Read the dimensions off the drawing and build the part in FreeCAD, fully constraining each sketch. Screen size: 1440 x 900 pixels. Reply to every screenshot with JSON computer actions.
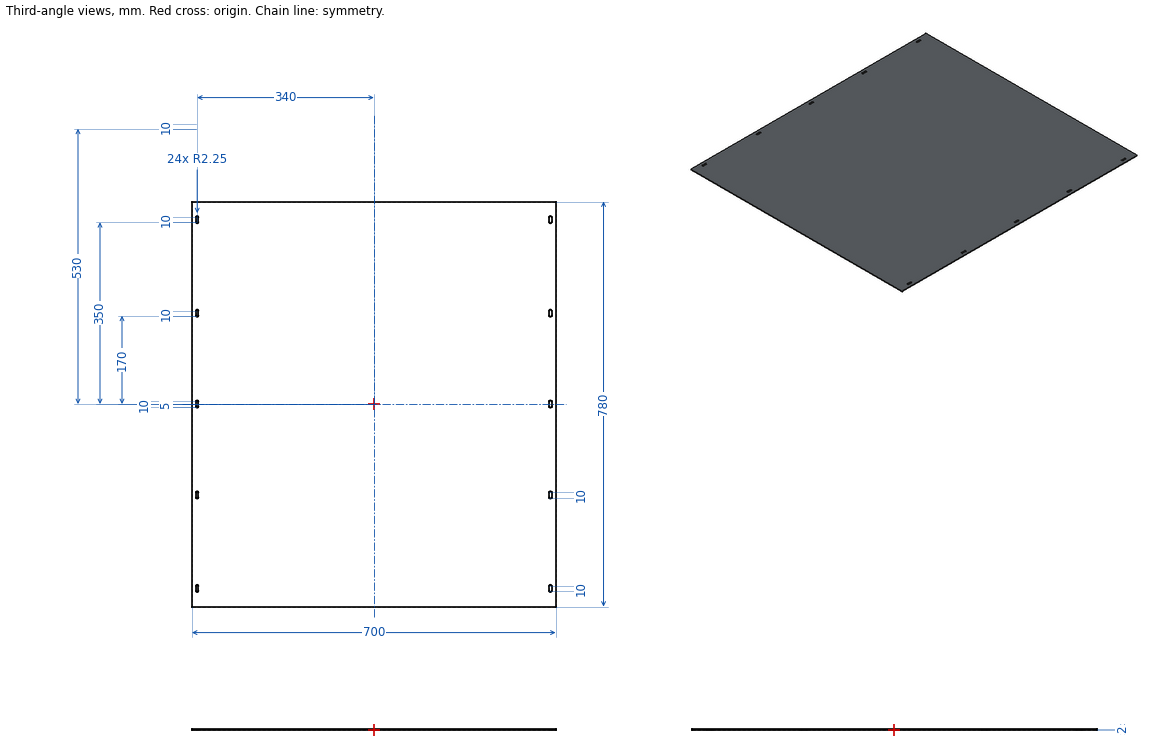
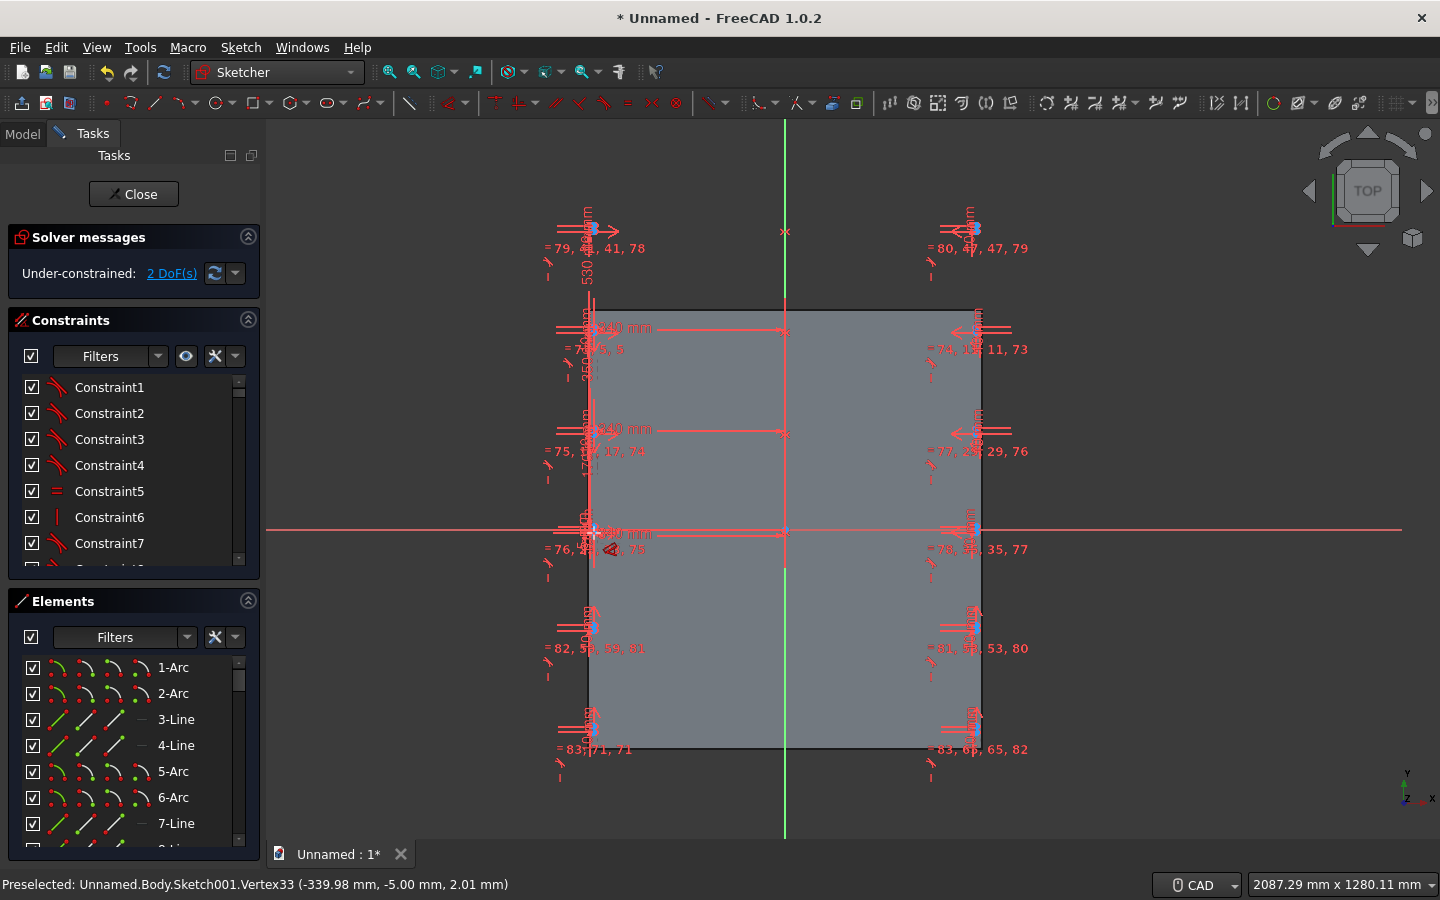
{"action": "scroll", "coordinate": [594, 232], "scroll_direction": "up", "scroll_amount": 12}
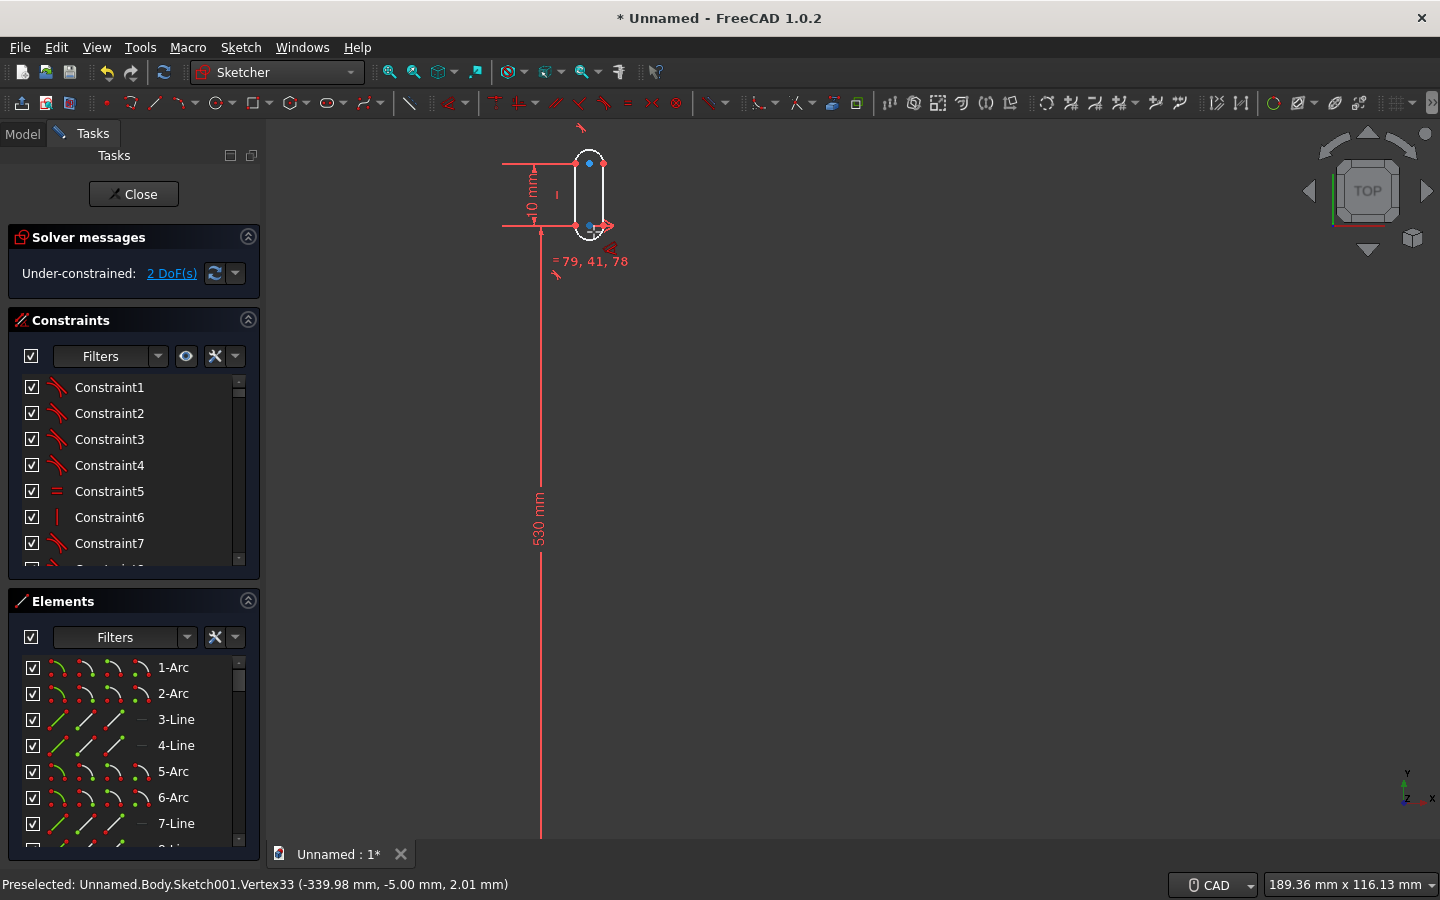
{"action": "left_click", "coordinate": [589, 226]}
{"action": "left_click", "coordinate": [932, 192]}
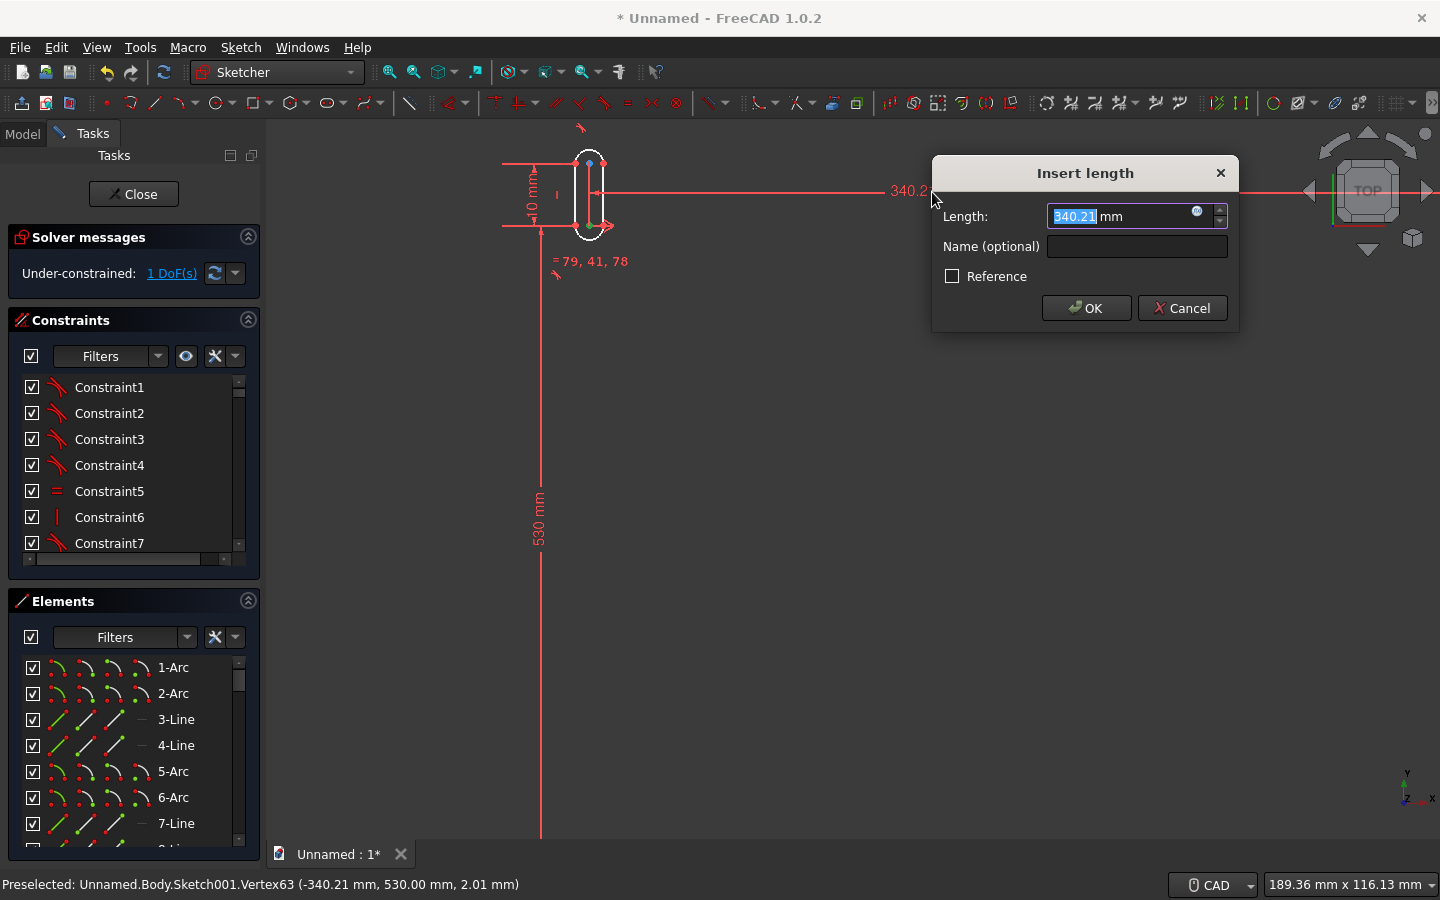
{"action": "type", "text": "340"}
{"action": "key", "text": "Return"}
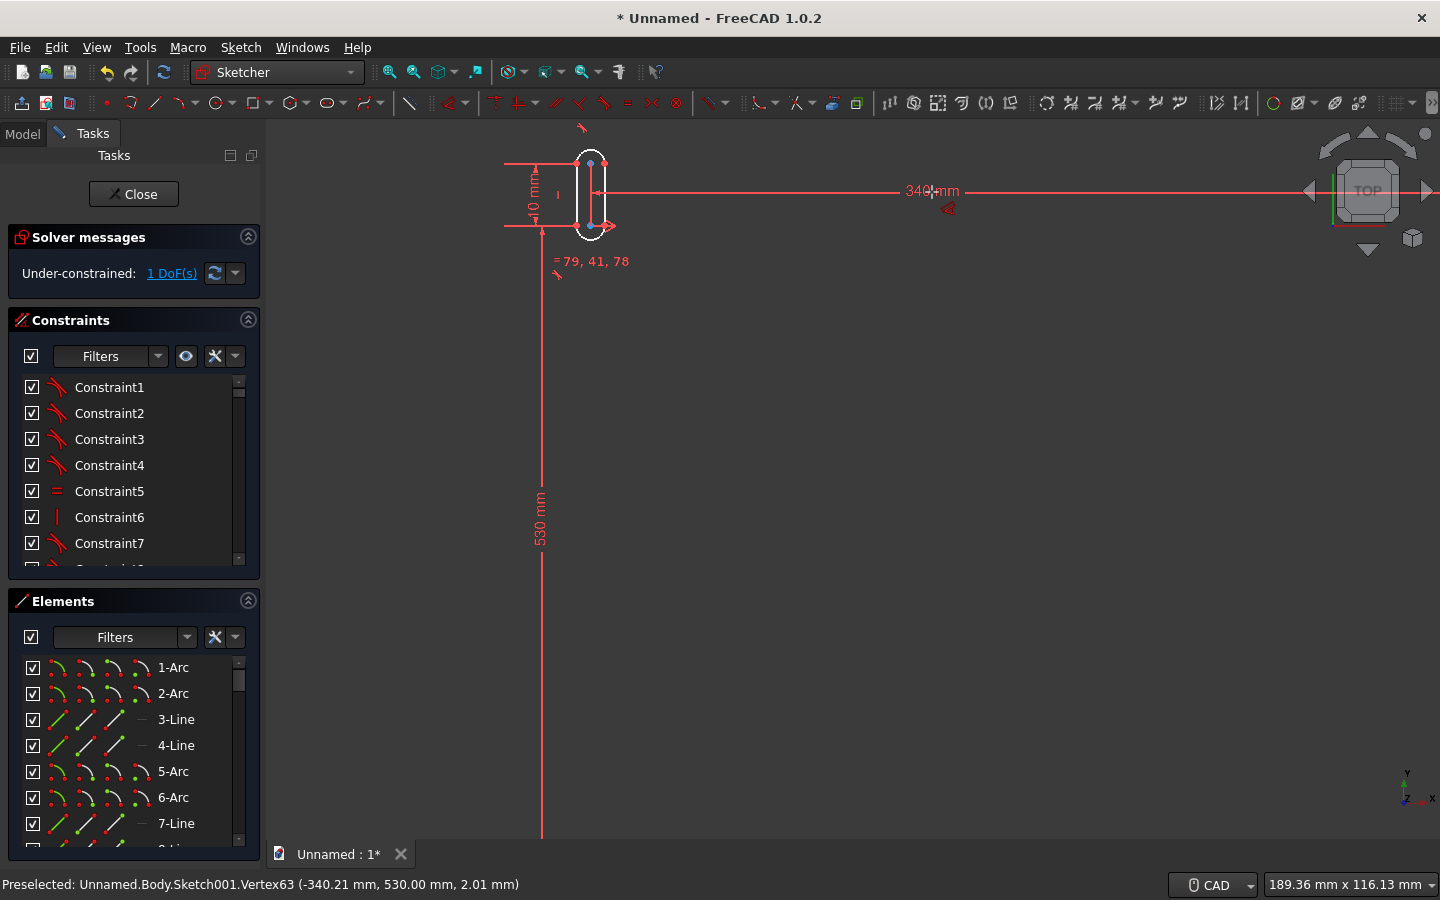
{"action": "scroll", "coordinate": [594, 232], "scroll_direction": "down", "scroll_amount": 12}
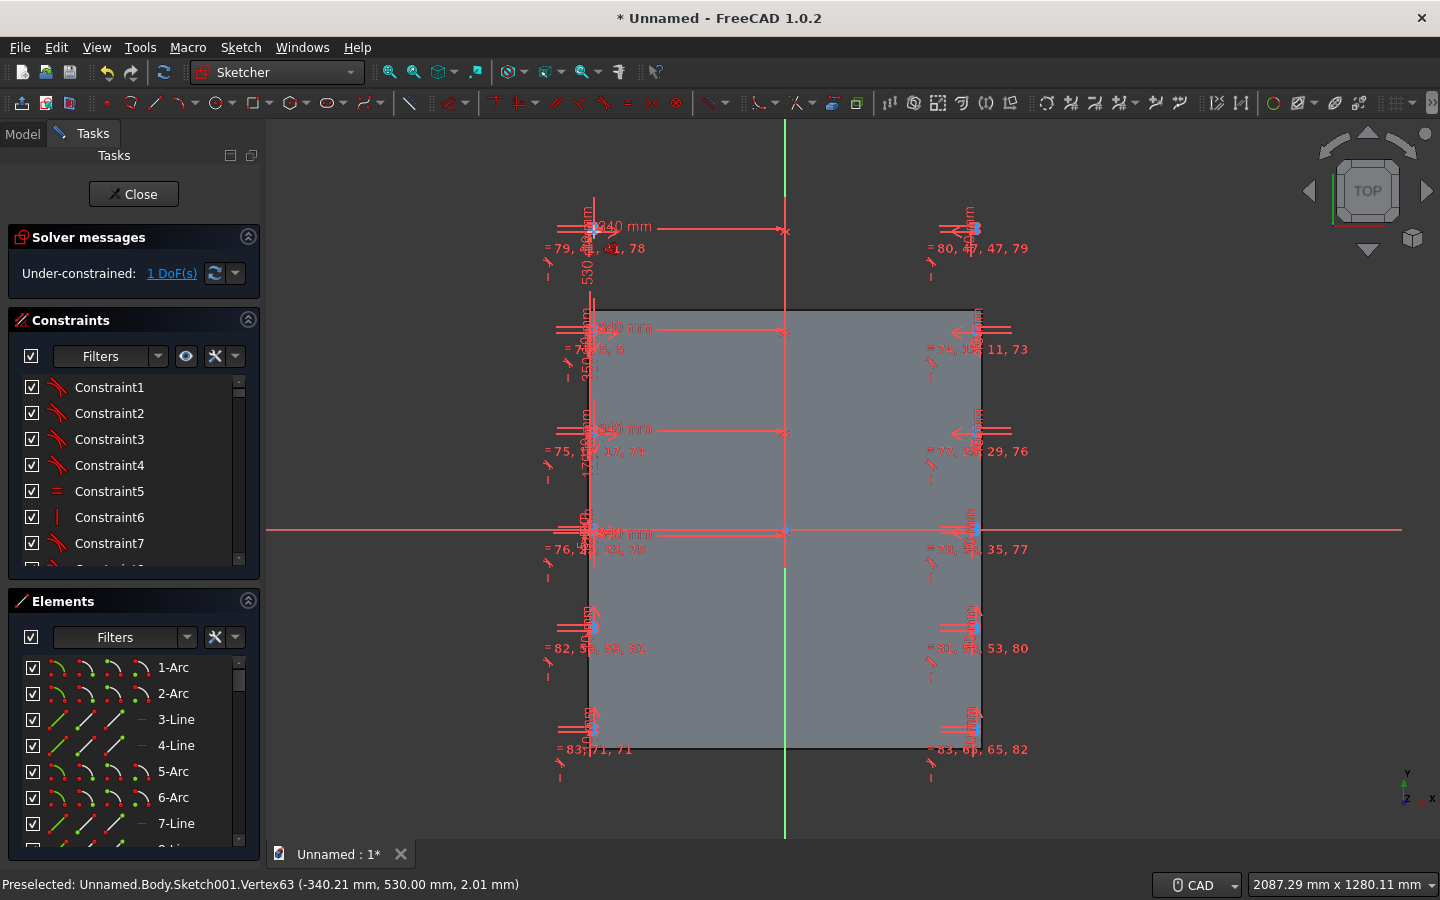
{"action": "scroll", "coordinate": [593, 334], "scroll_direction": "up", "scroll_amount": 18}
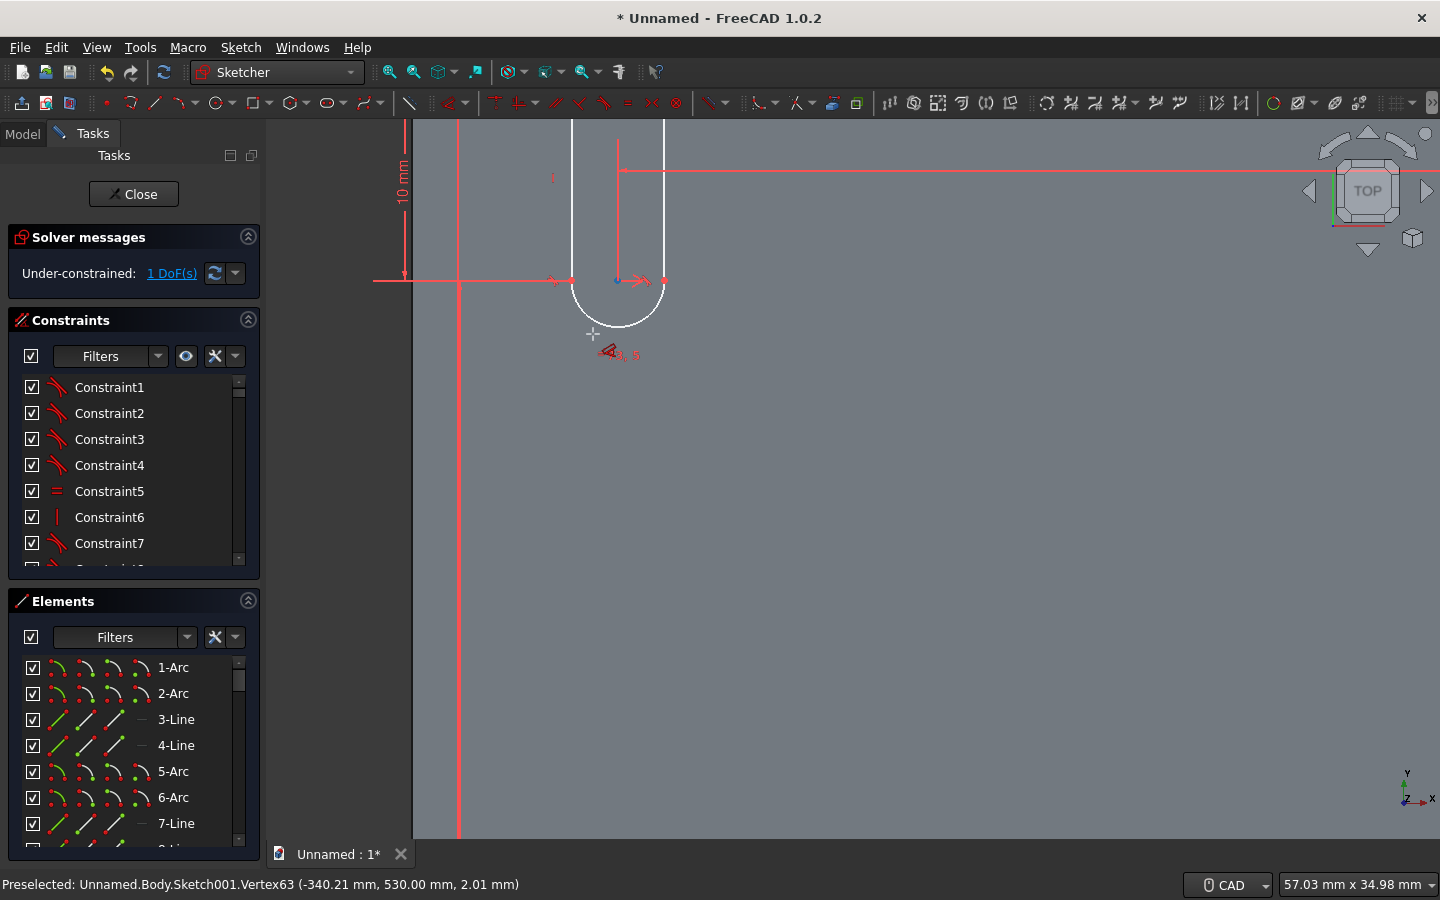
{"action": "left_click", "coordinate": [591, 318]}
{"action": "left_click", "coordinate": [572, 344]}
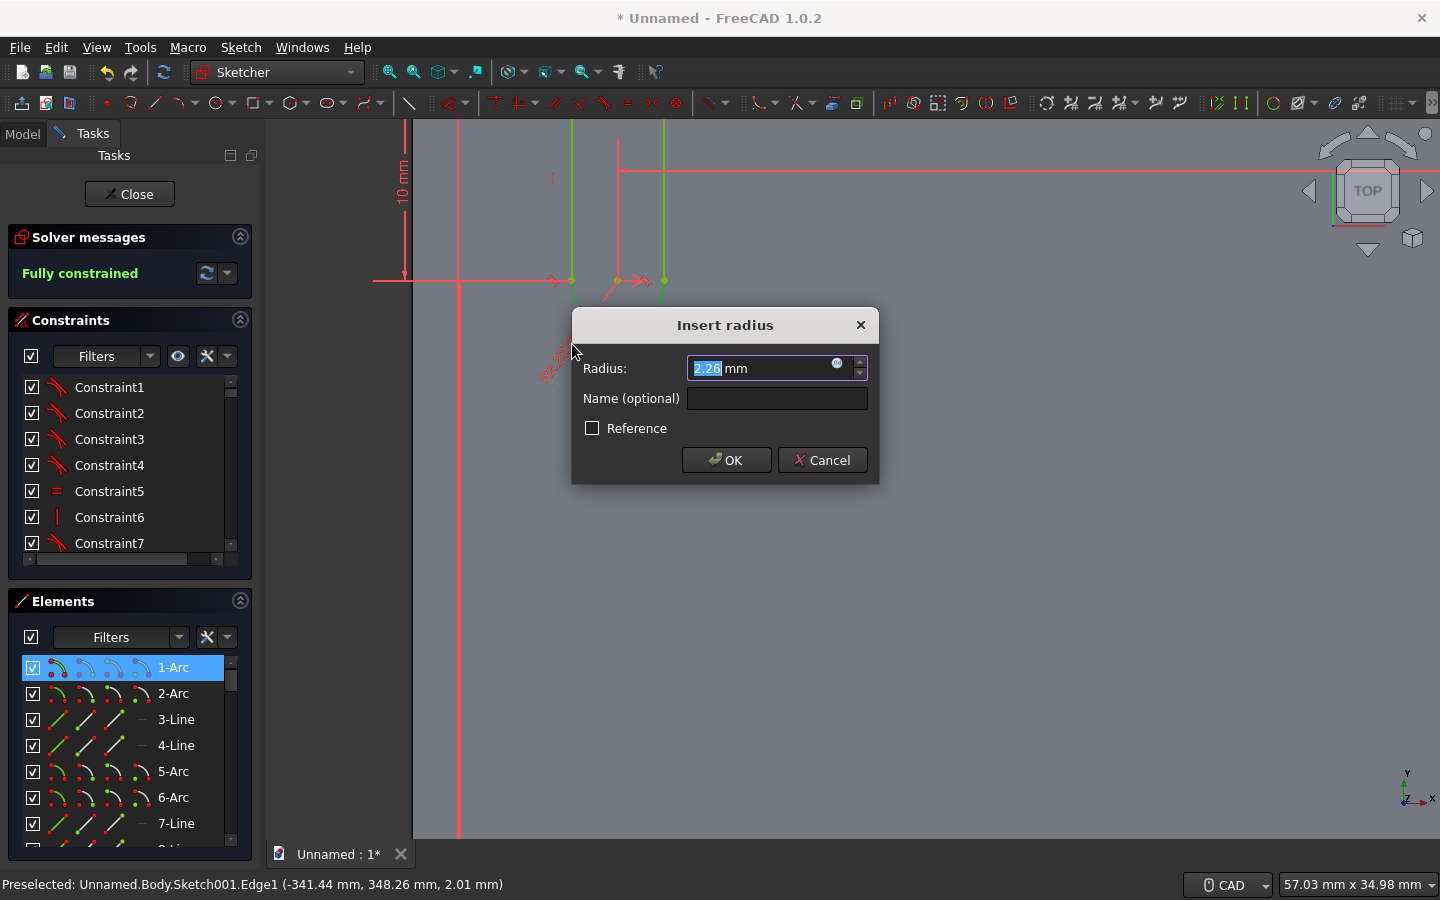
{"action": "type", "text": "2.25"}
{"action": "key", "text": "Return"}
{"action": "key", "text": "Escape"}